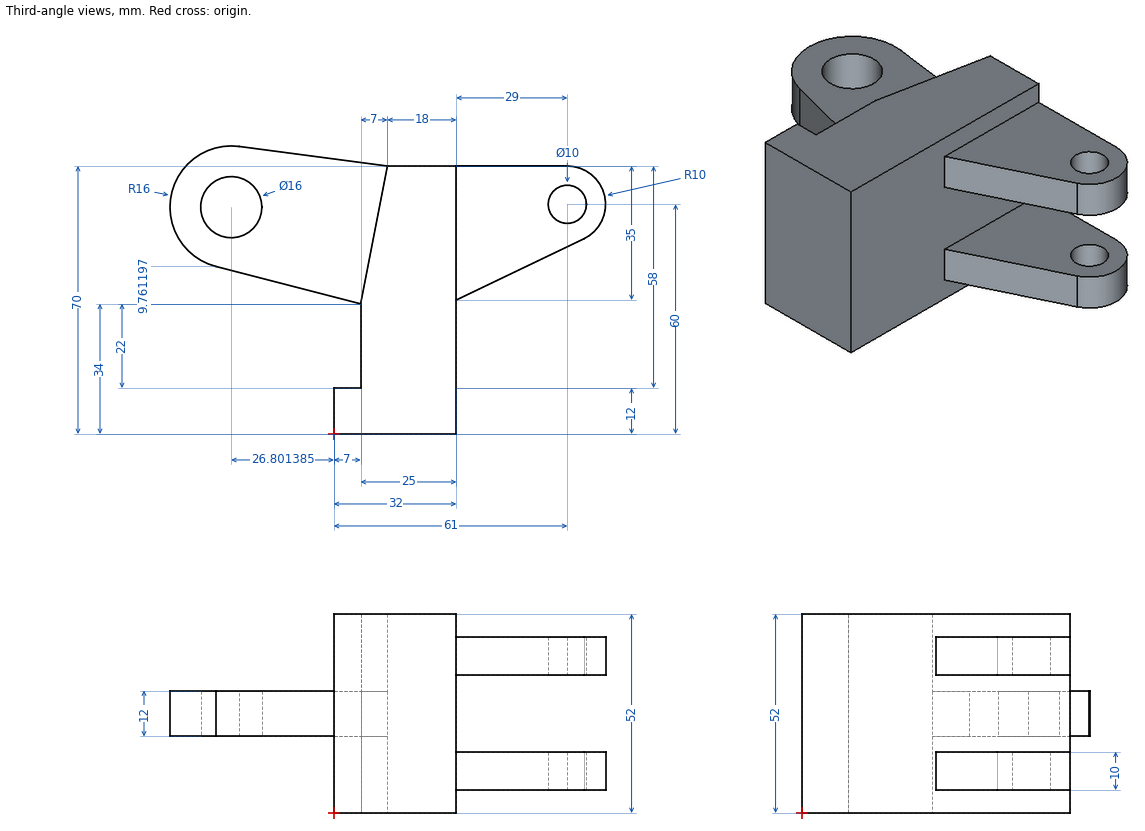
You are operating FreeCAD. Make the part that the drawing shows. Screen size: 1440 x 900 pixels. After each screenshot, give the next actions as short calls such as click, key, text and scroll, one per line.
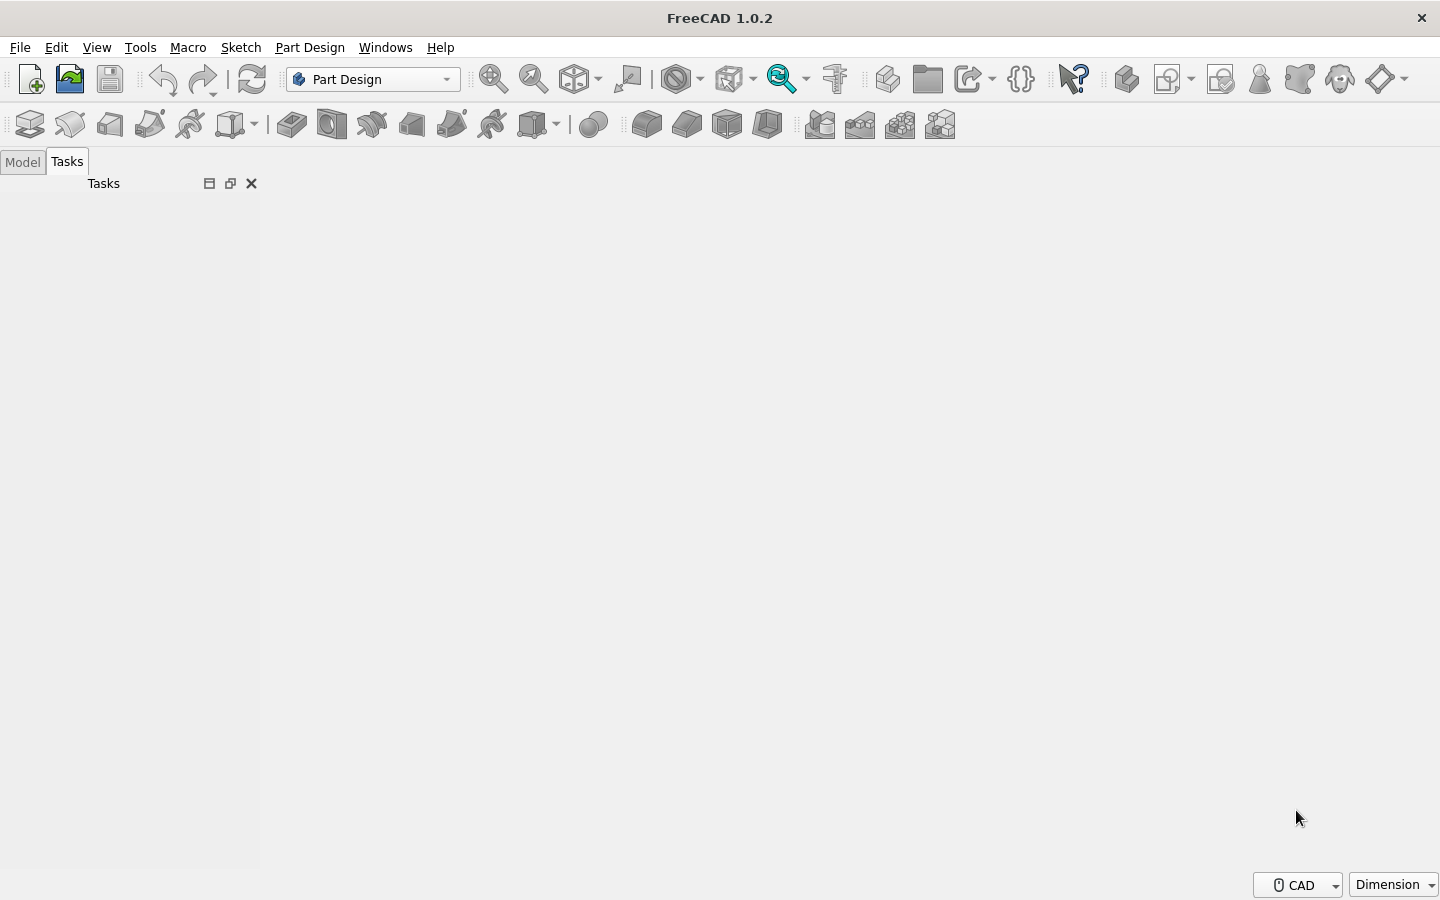
key(ctrl+n)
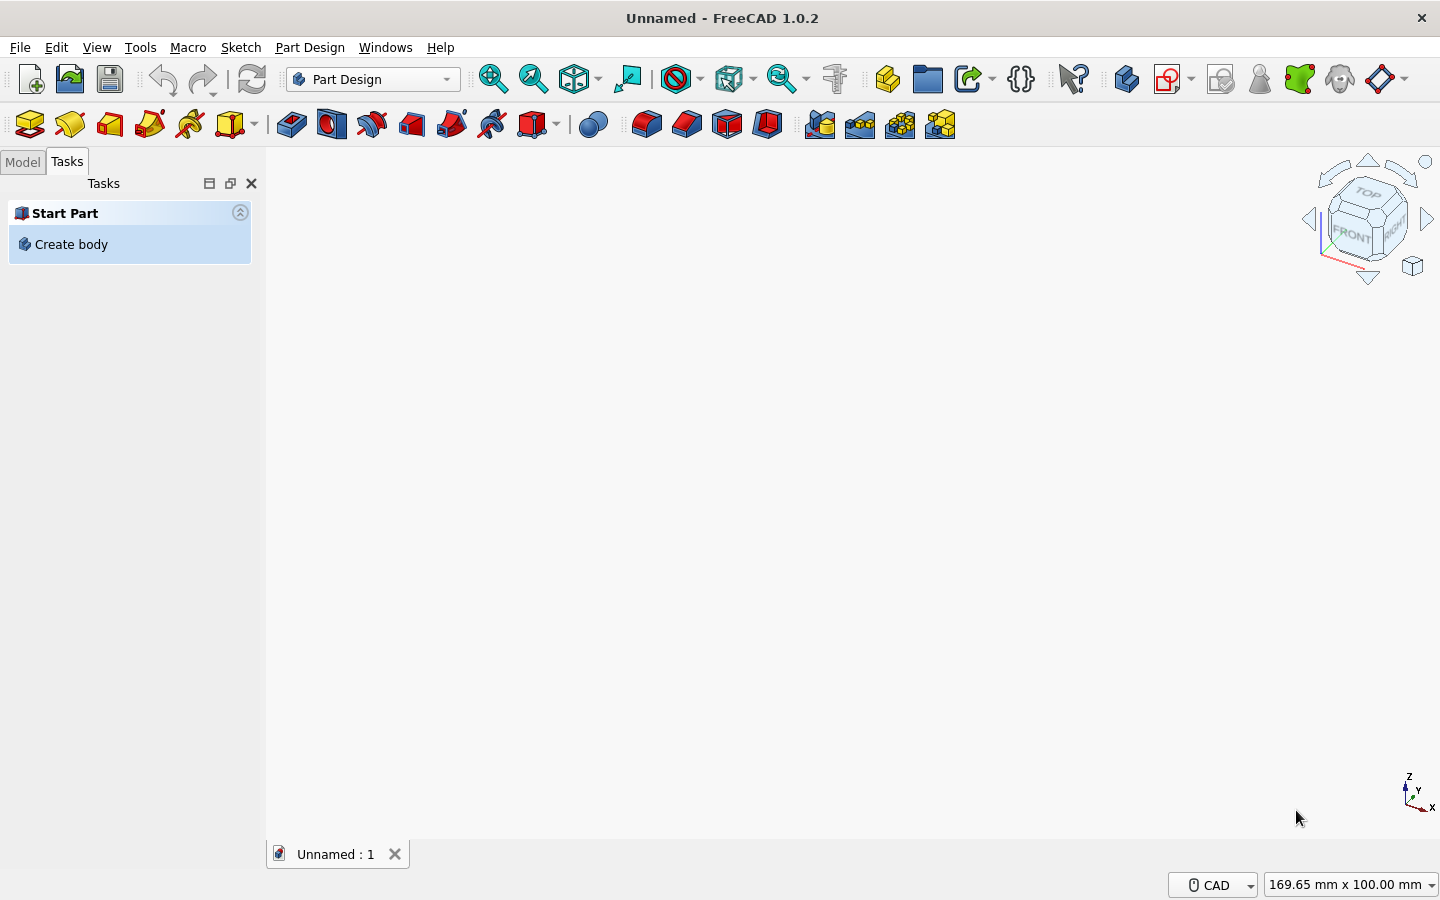
click(1168, 80)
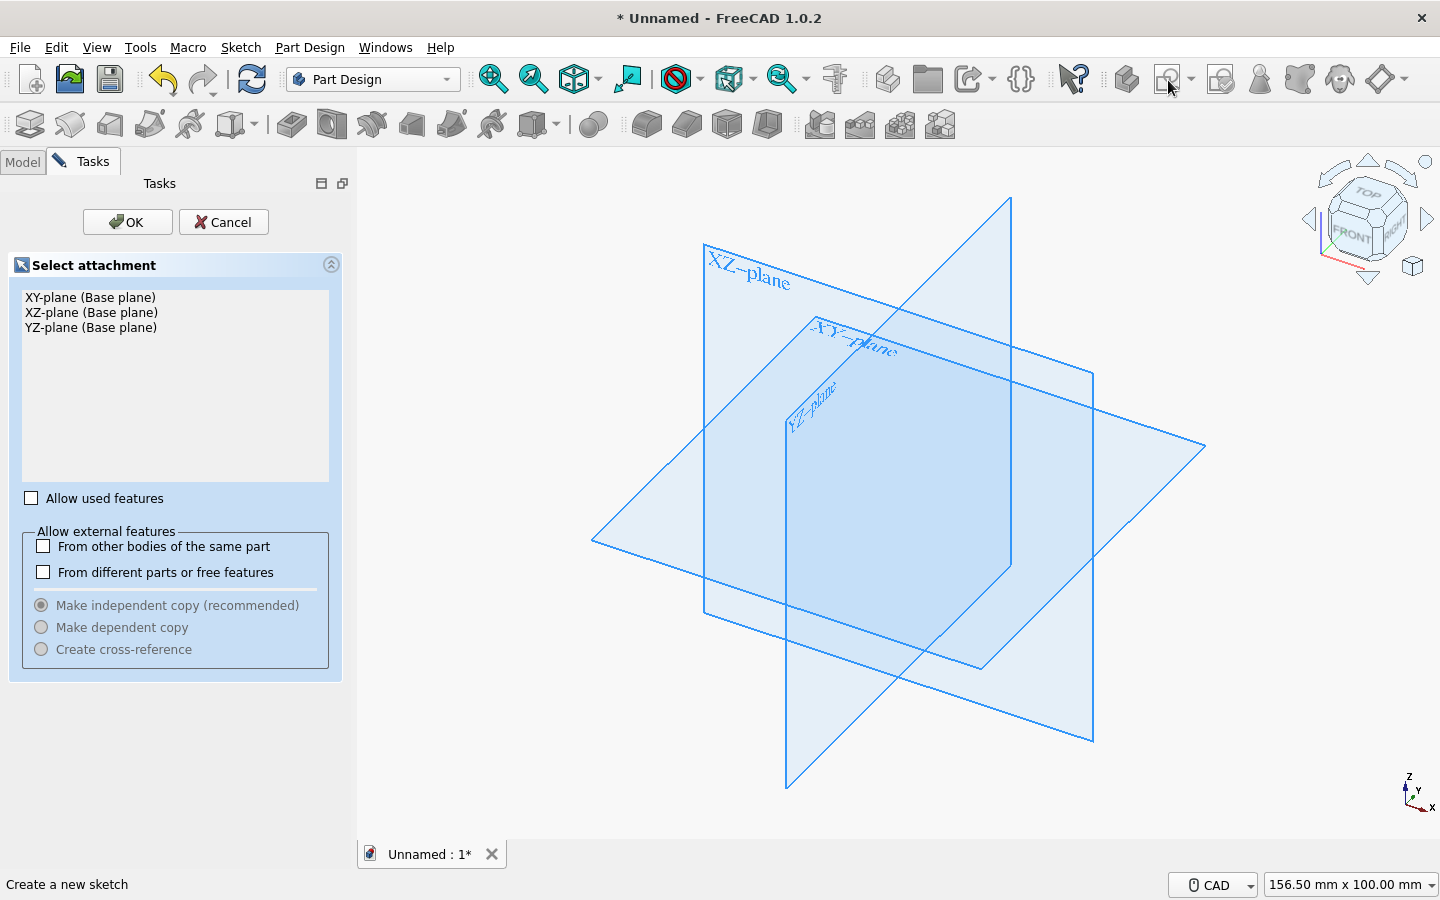
click(82, 298)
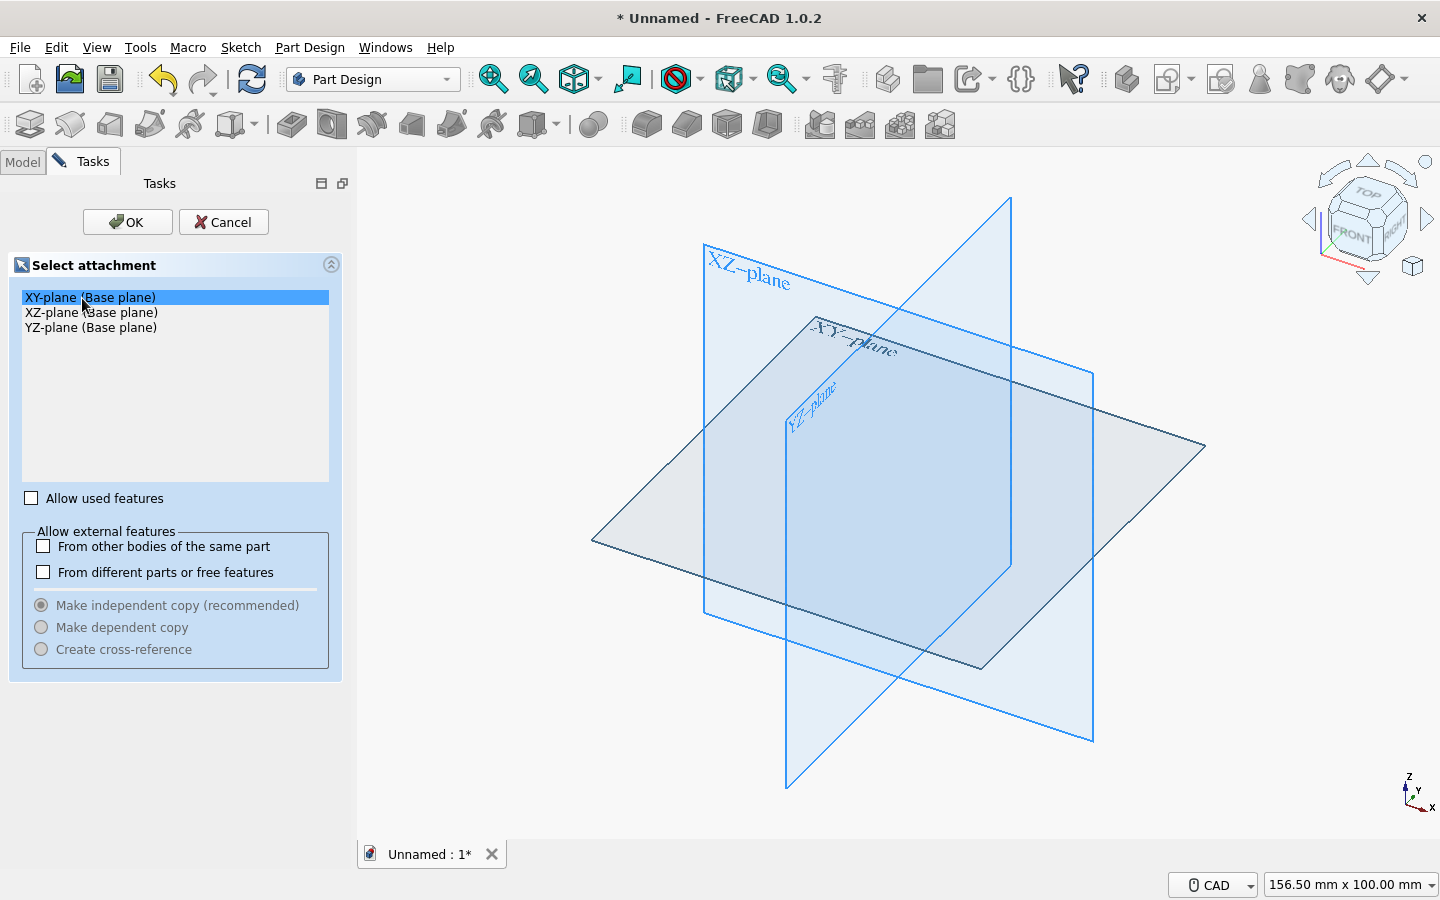
click(128, 222)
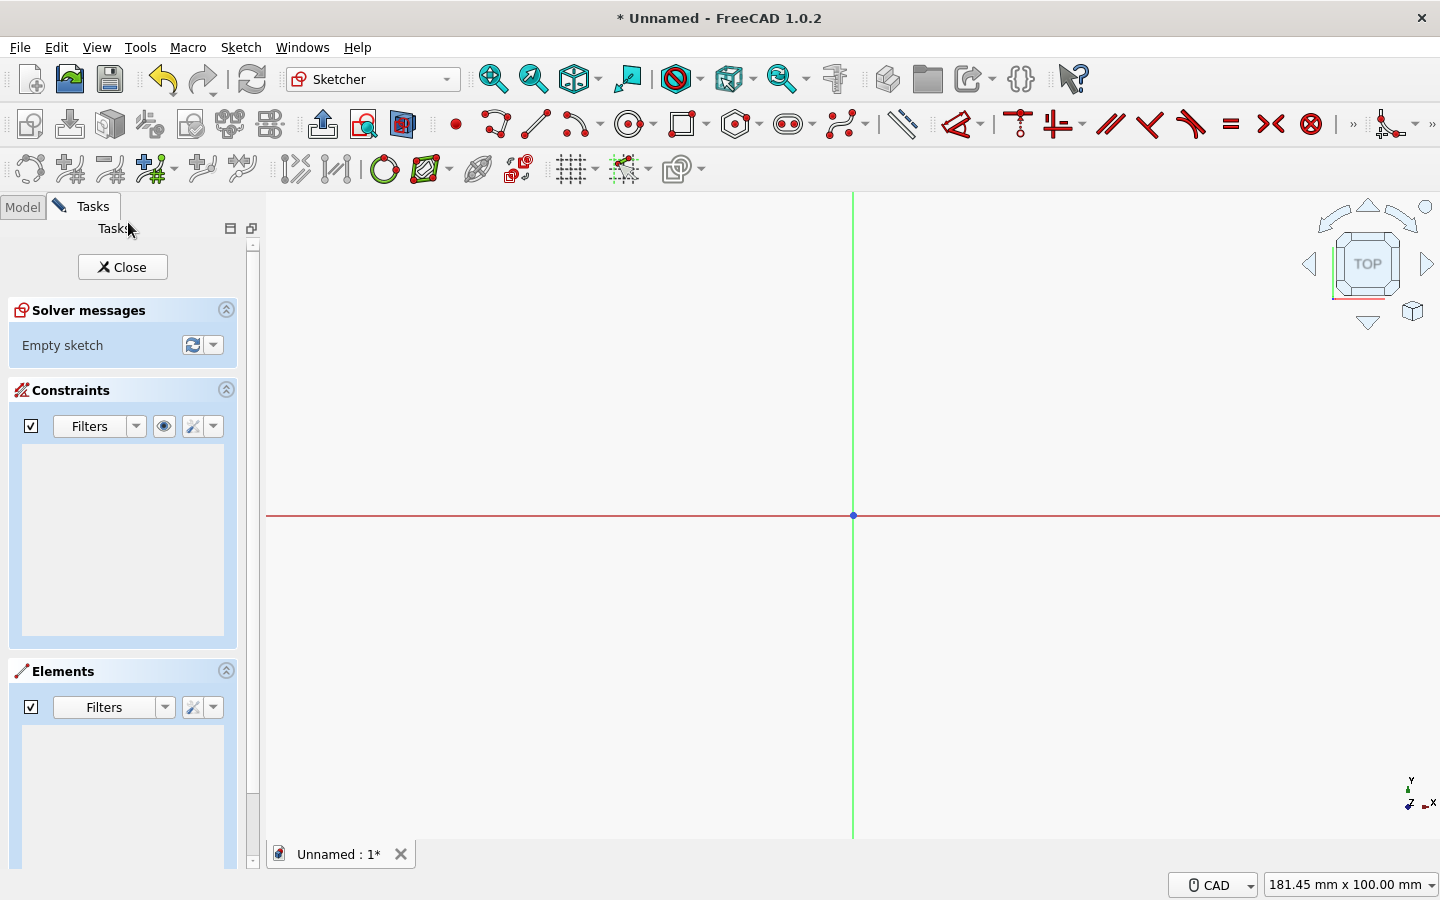
scroll(1031, 460, up, 6)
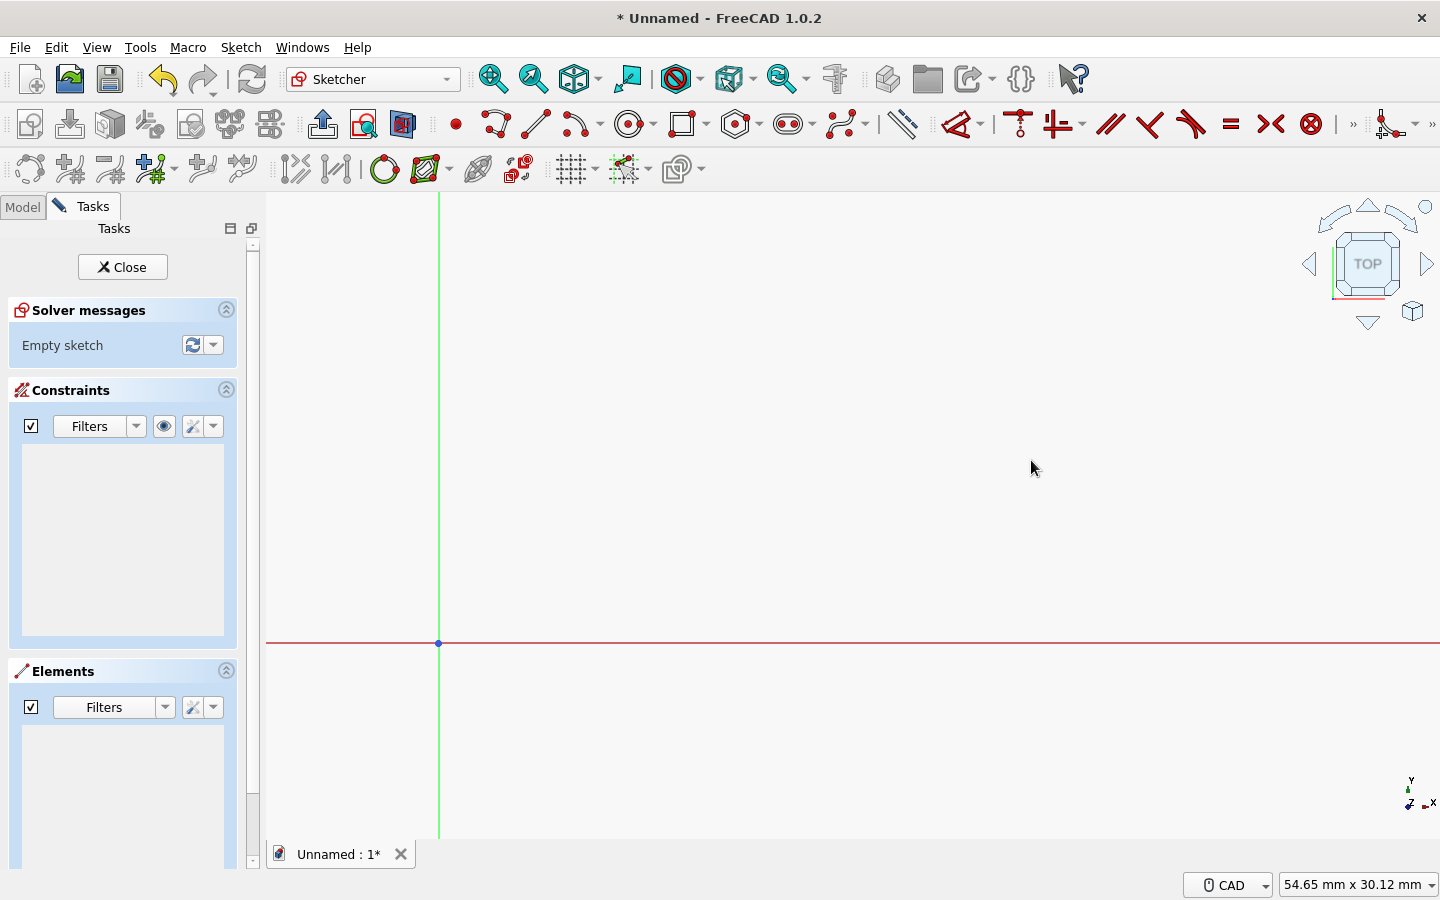
click(682, 124)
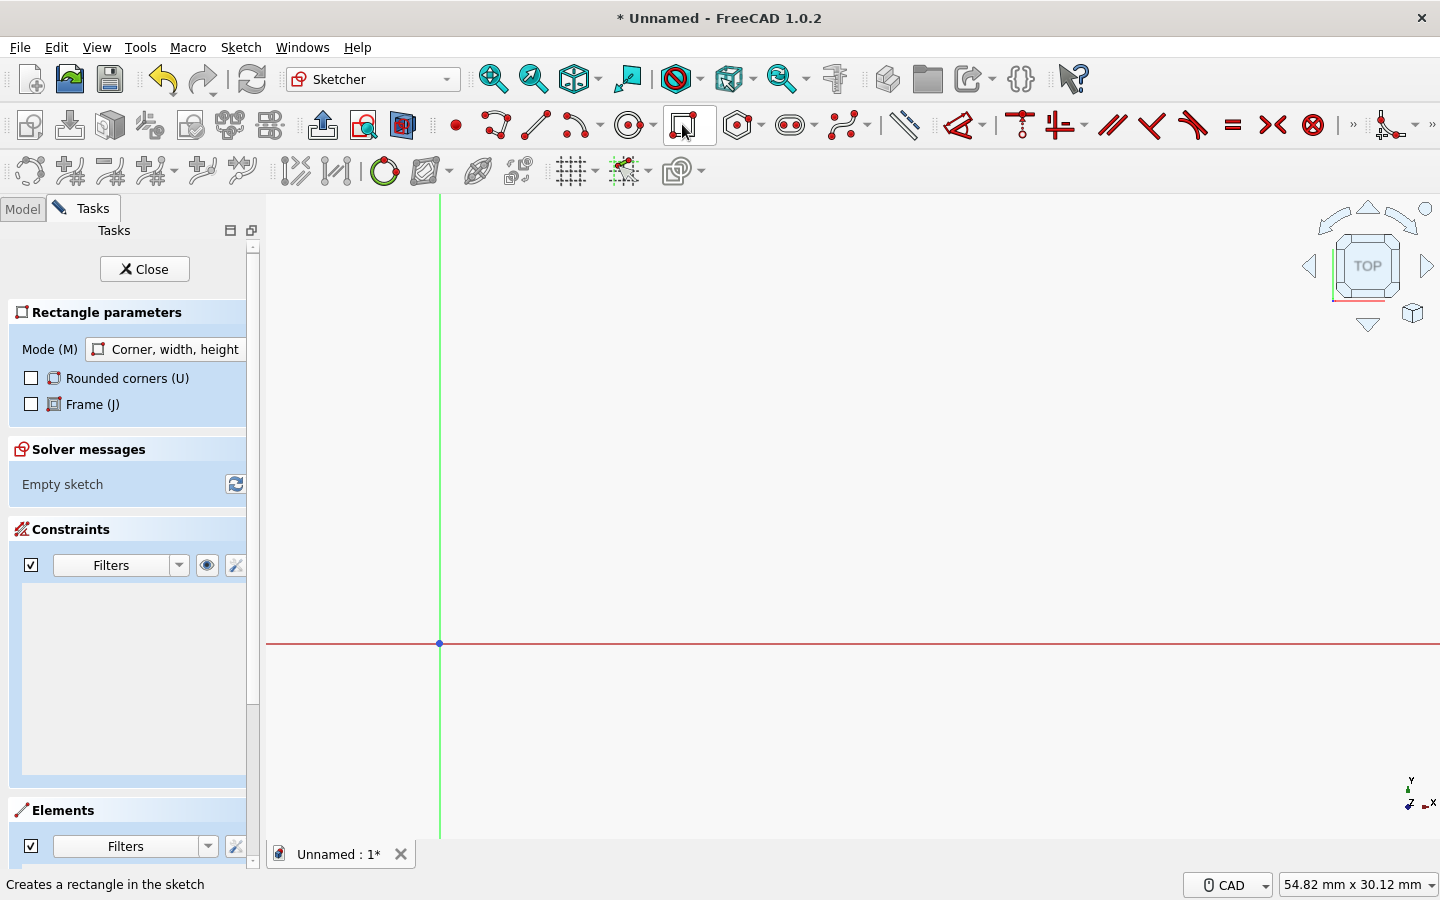
click(440, 644)
move(1125, 387)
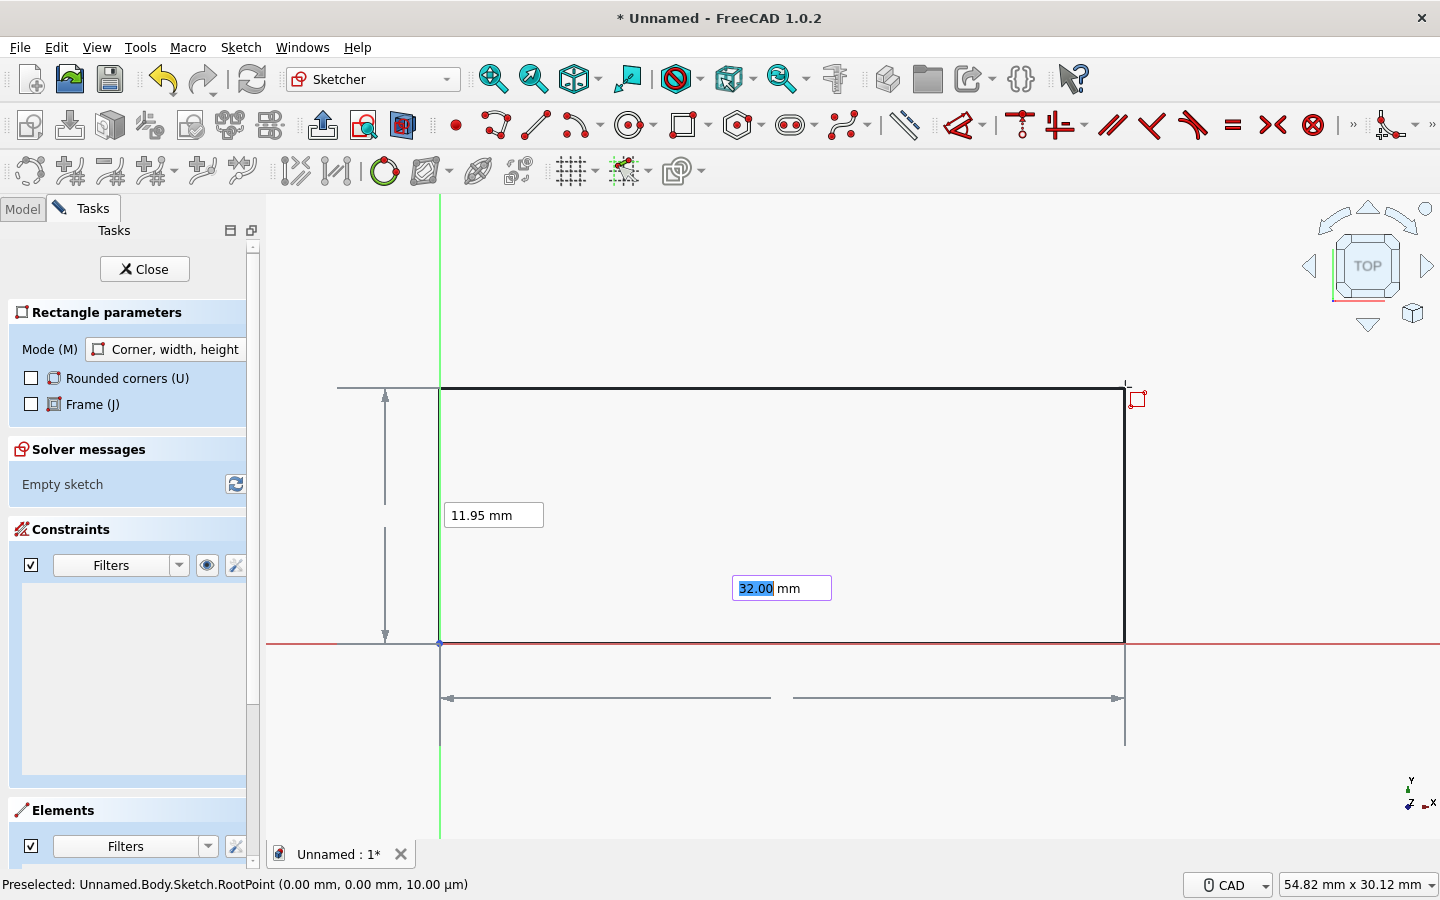
text(32)
key(Tab)
text(12)
key(Return)
key(Escape)